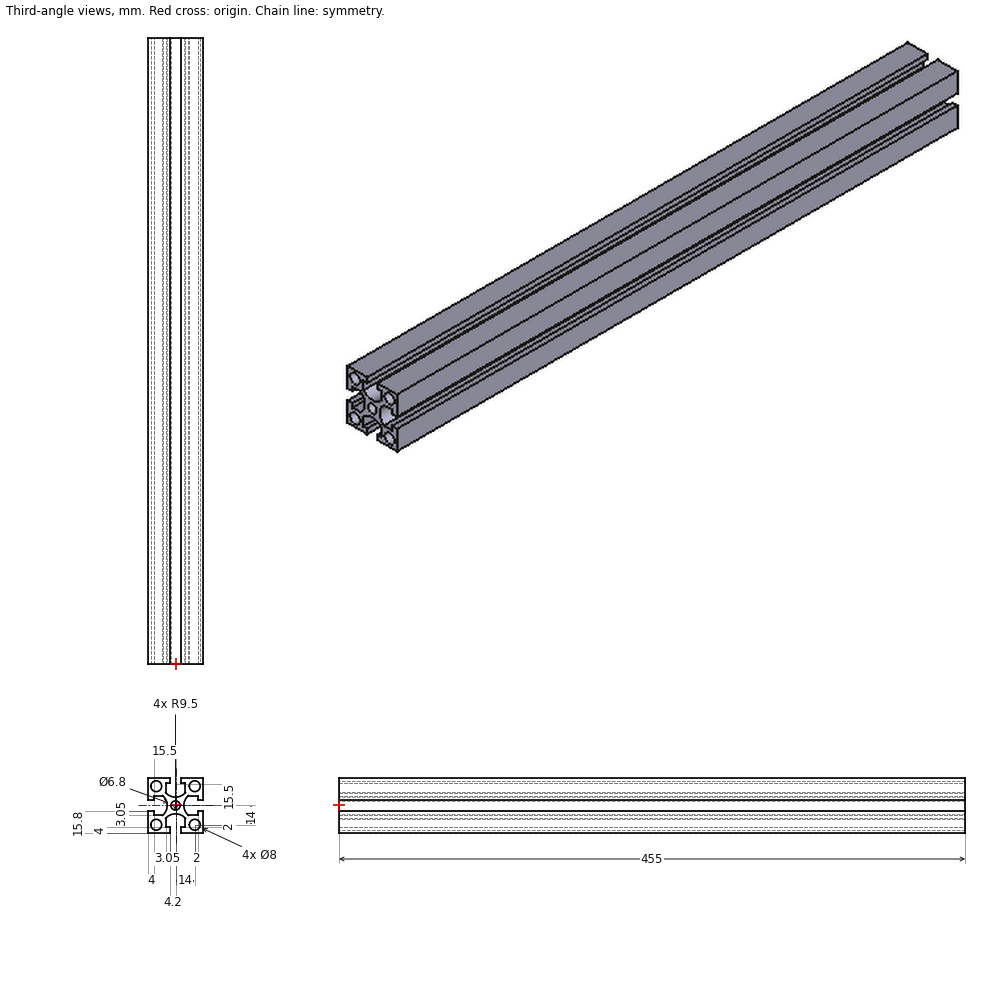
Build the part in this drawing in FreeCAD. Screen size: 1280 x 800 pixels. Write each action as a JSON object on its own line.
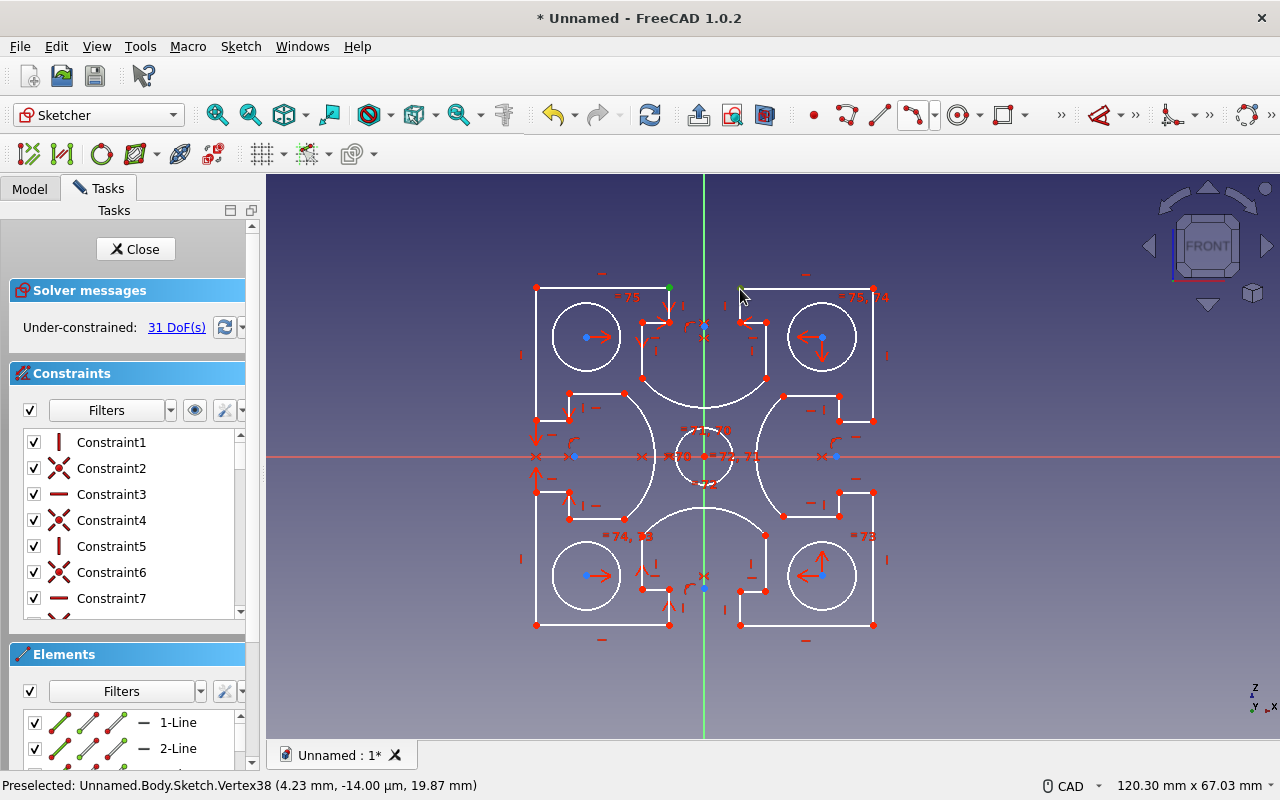
{"action": "left_click", "coordinate": [704, 675]}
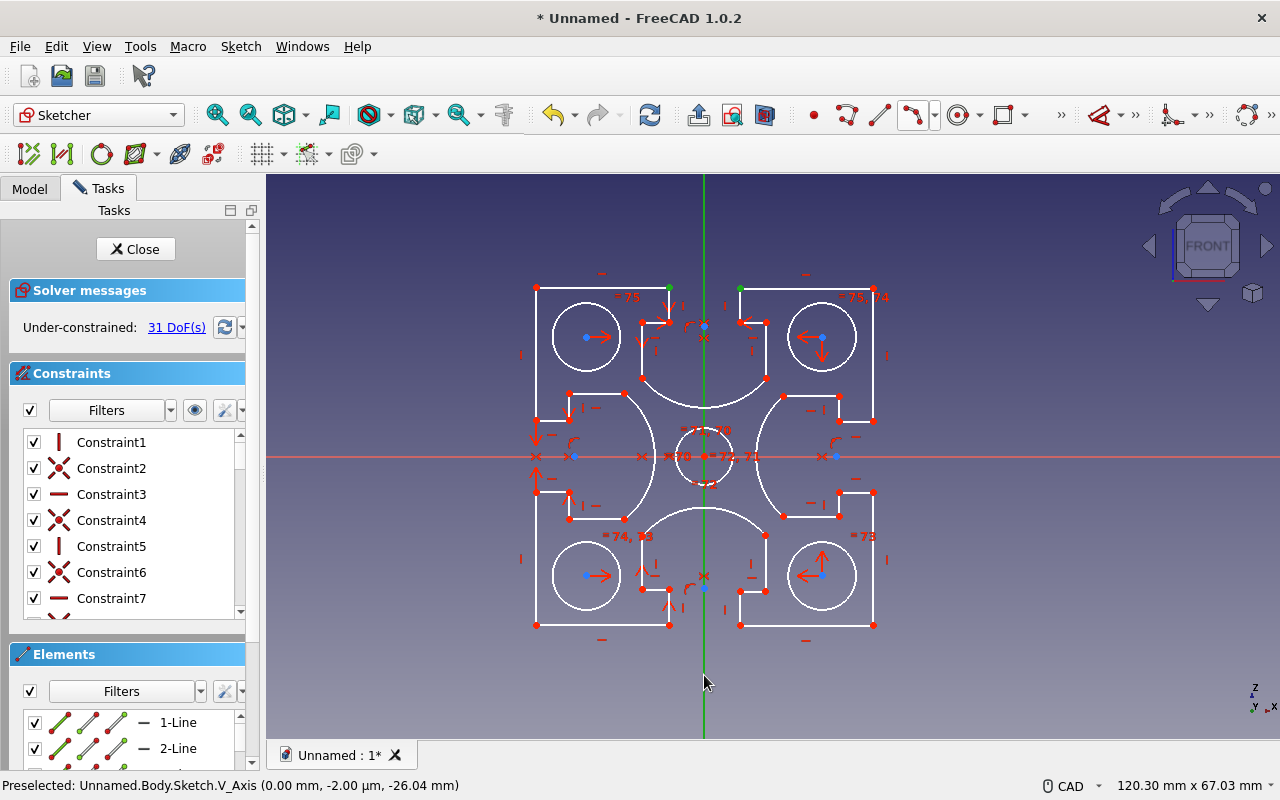
{"action": "key", "text": "s"}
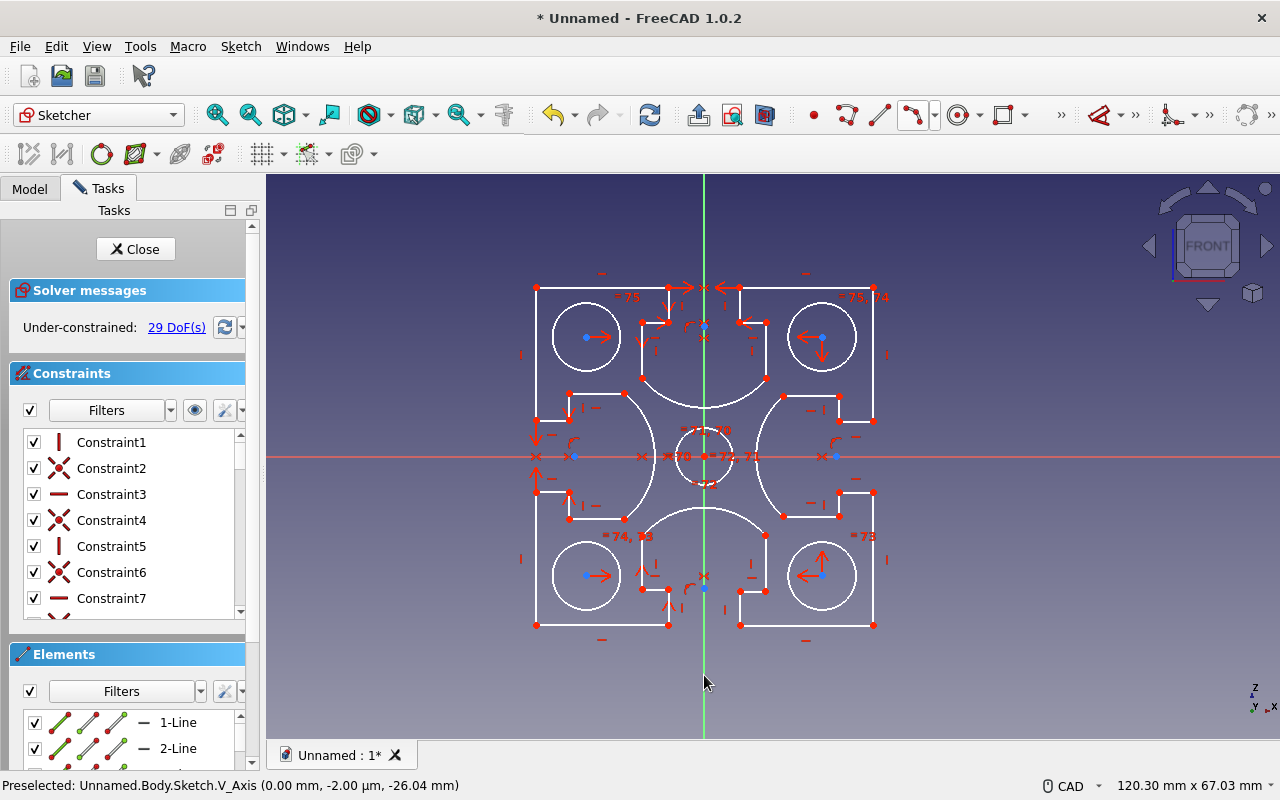
{"action": "left_click", "coordinate": [536, 421]}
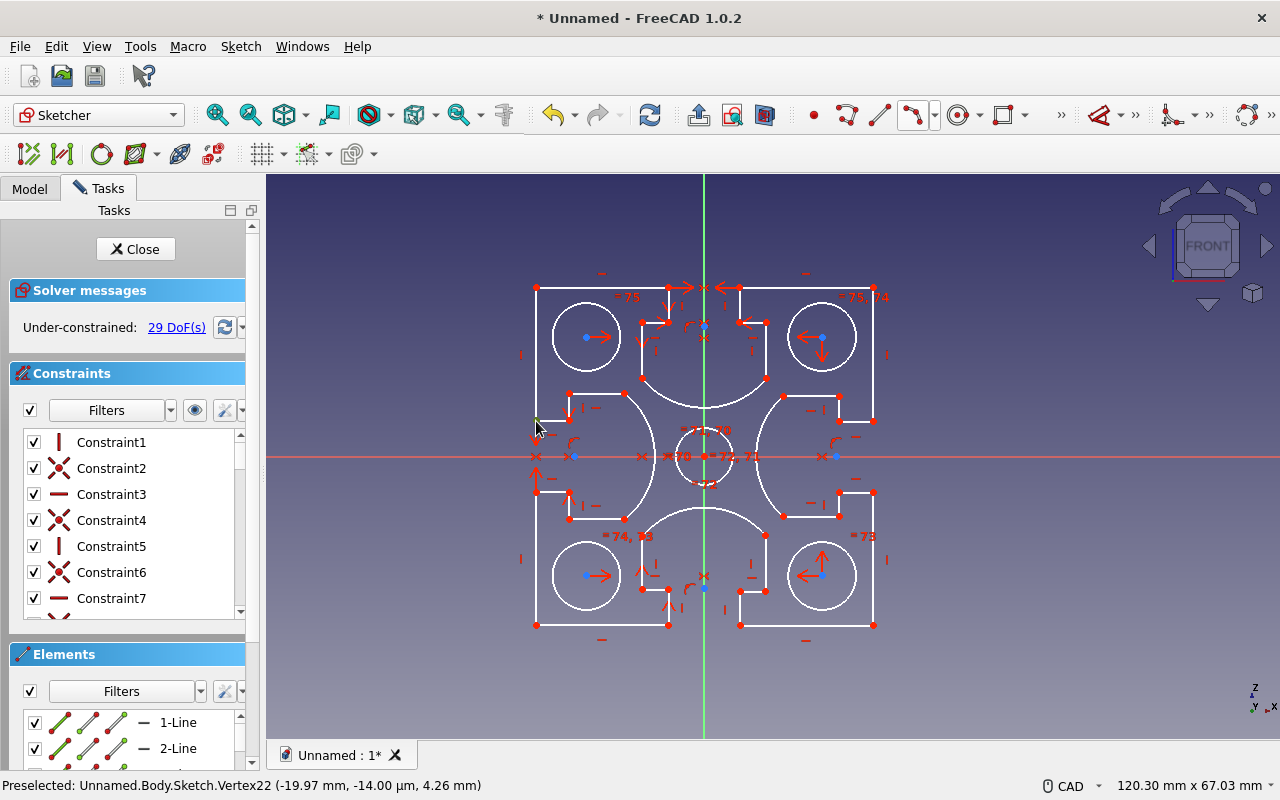
{"action": "left_click", "coordinate": [873, 422]}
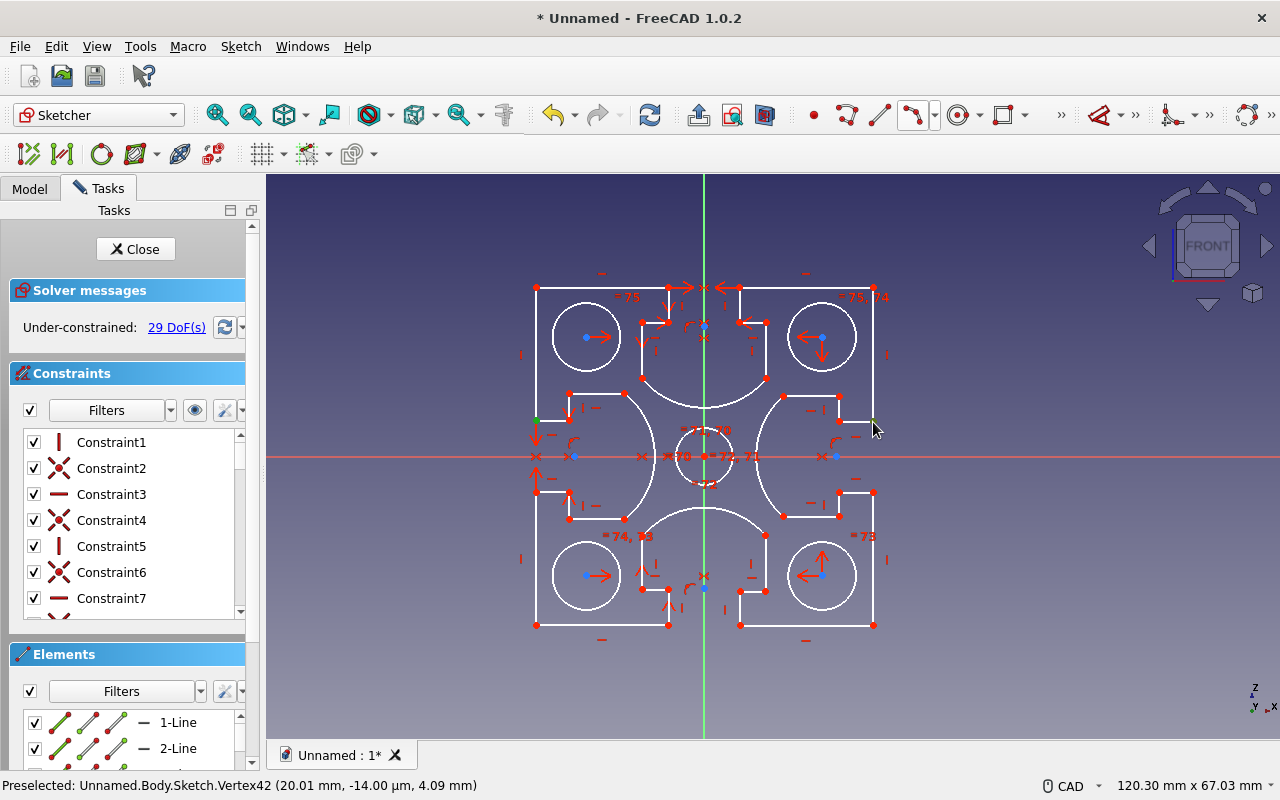
{"action": "left_click", "coordinate": [704, 675]}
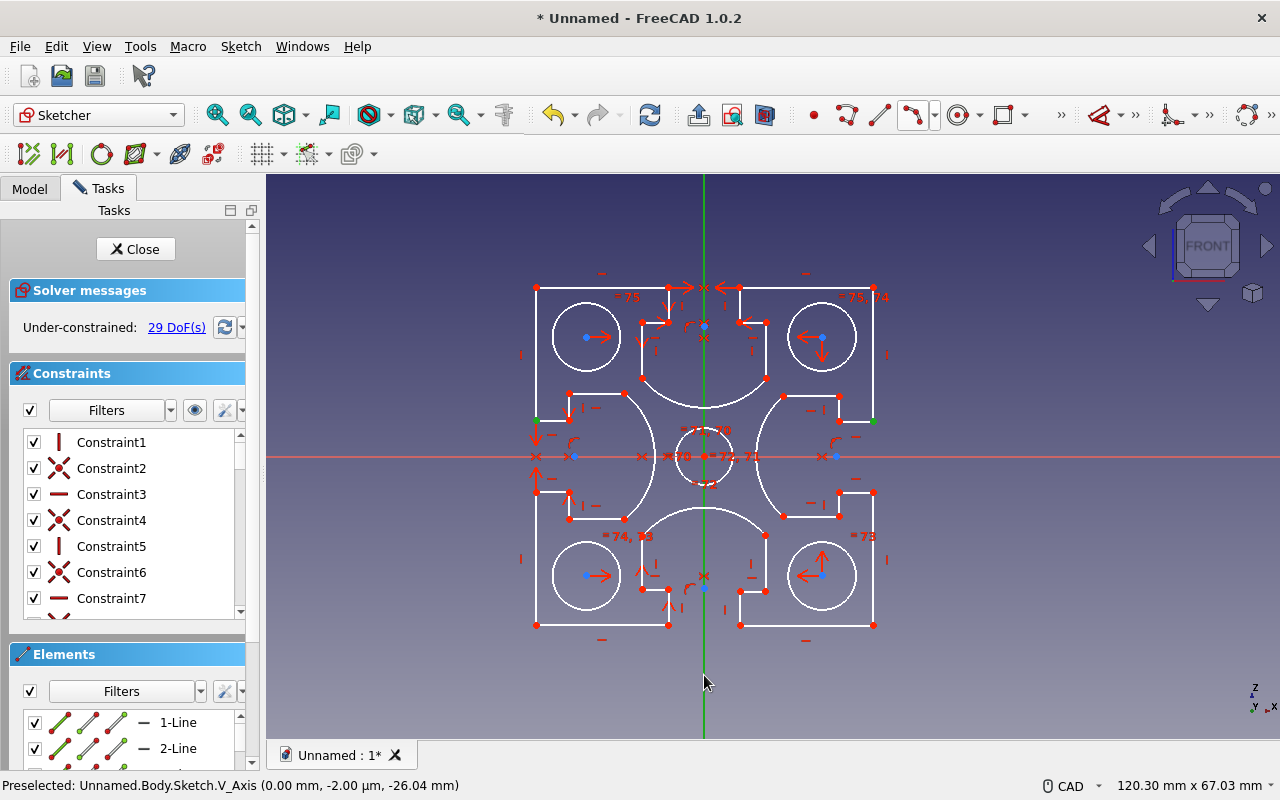
{"action": "key", "text": "s"}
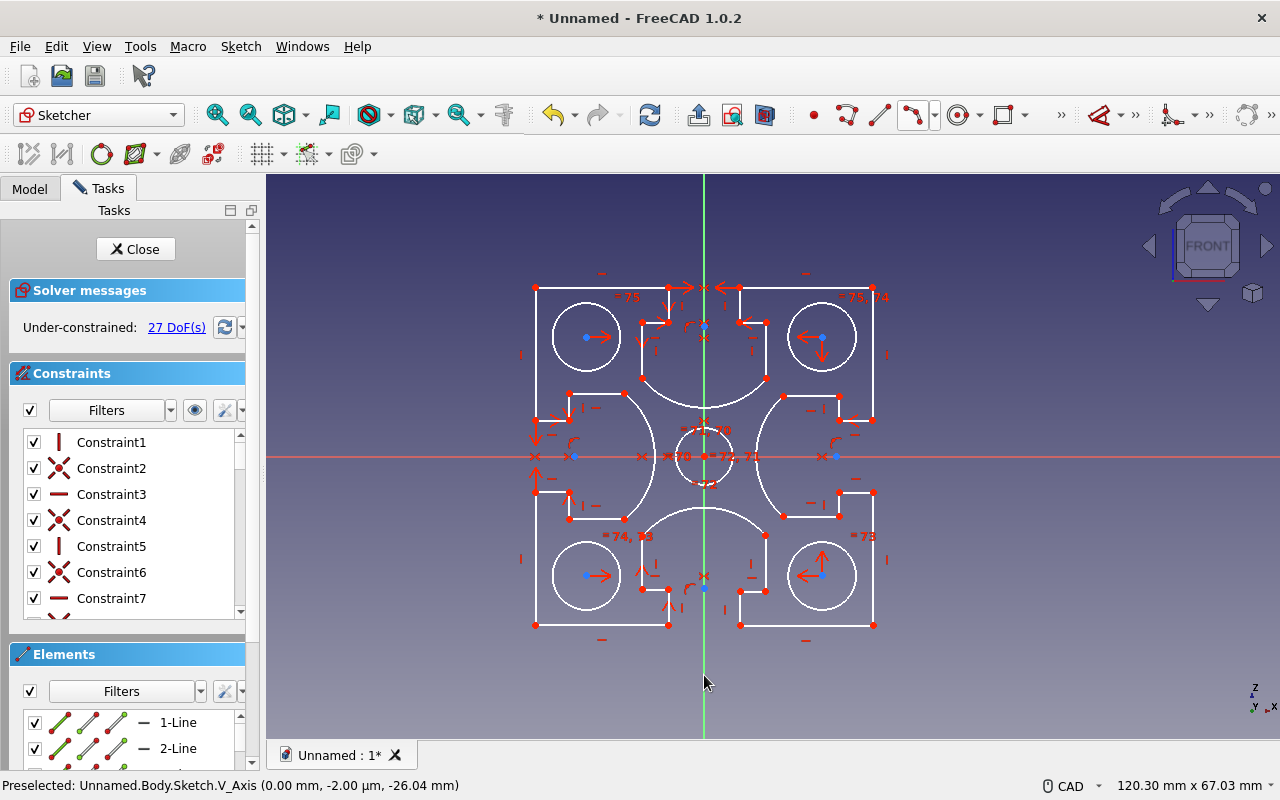
{"action": "left_click", "coordinate": [569, 394]}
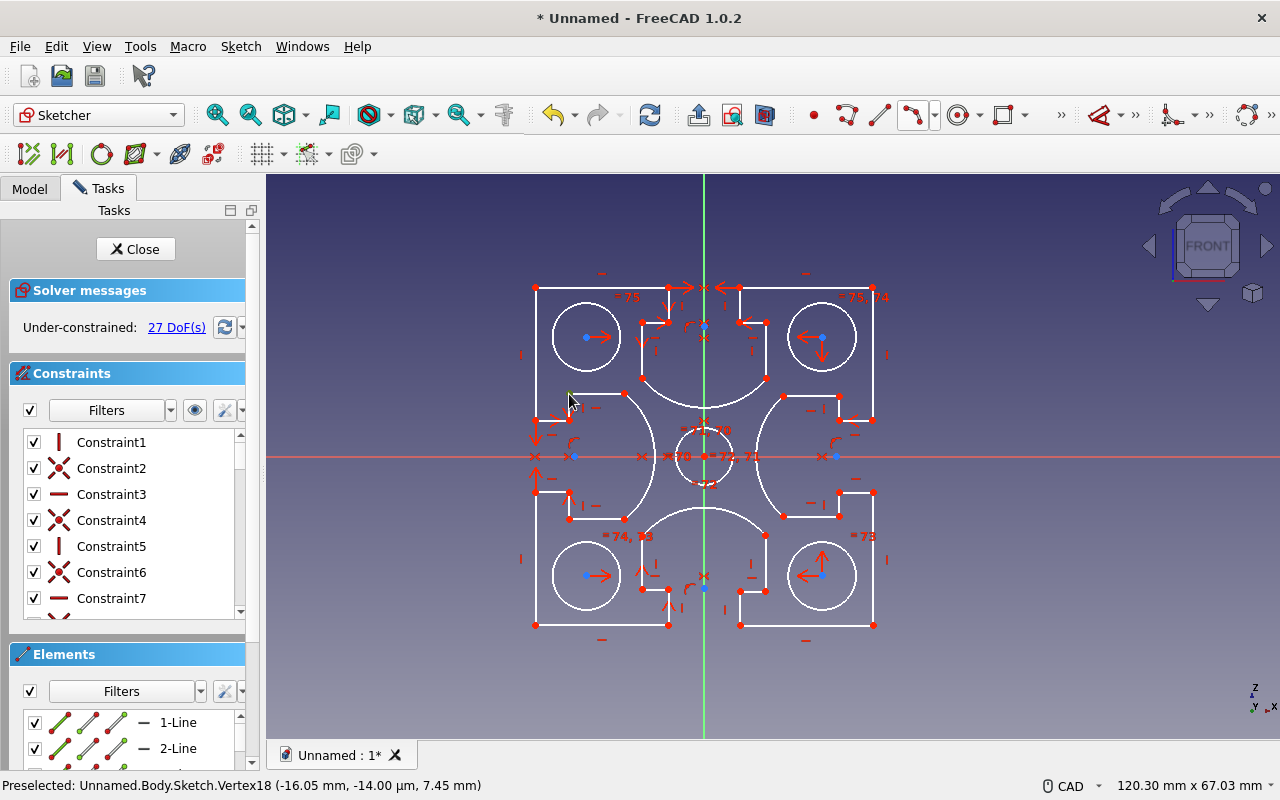
{"action": "left_click", "coordinate": [839, 396]}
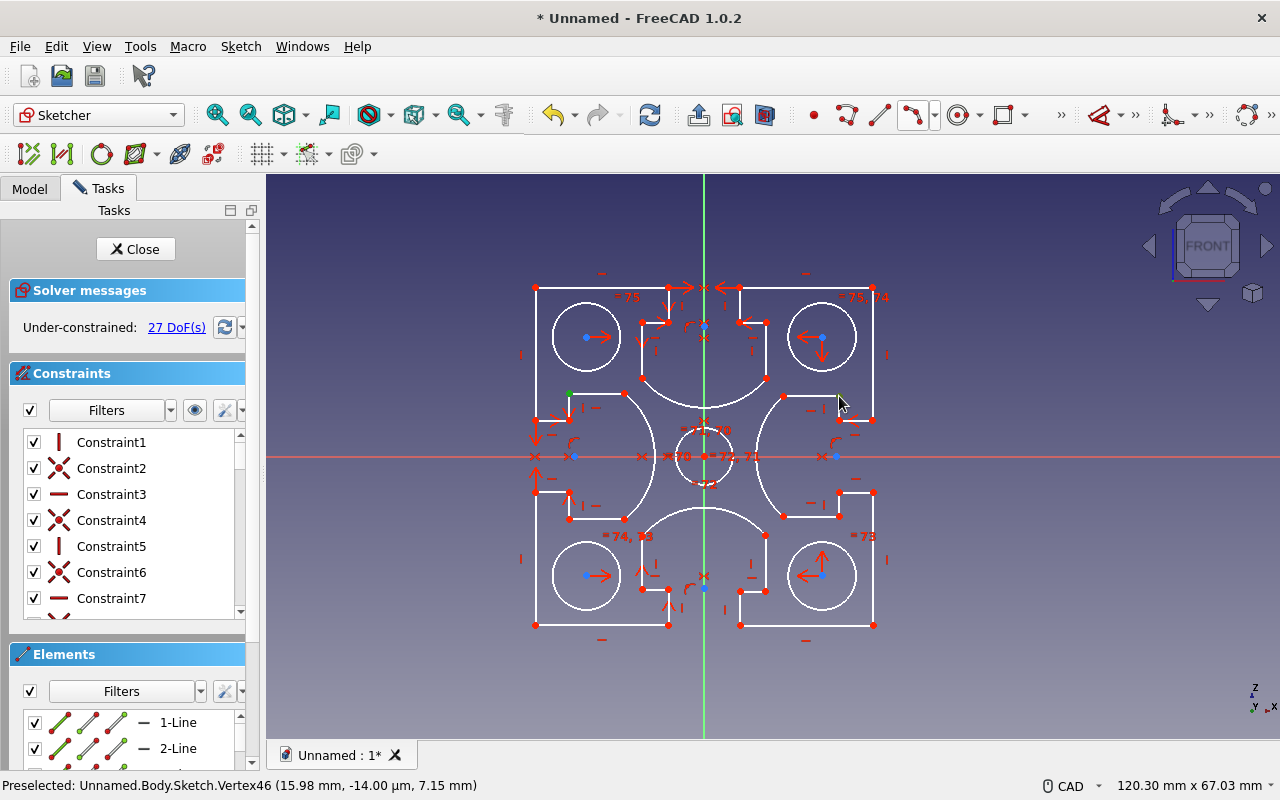
{"action": "left_click", "coordinate": [704, 675]}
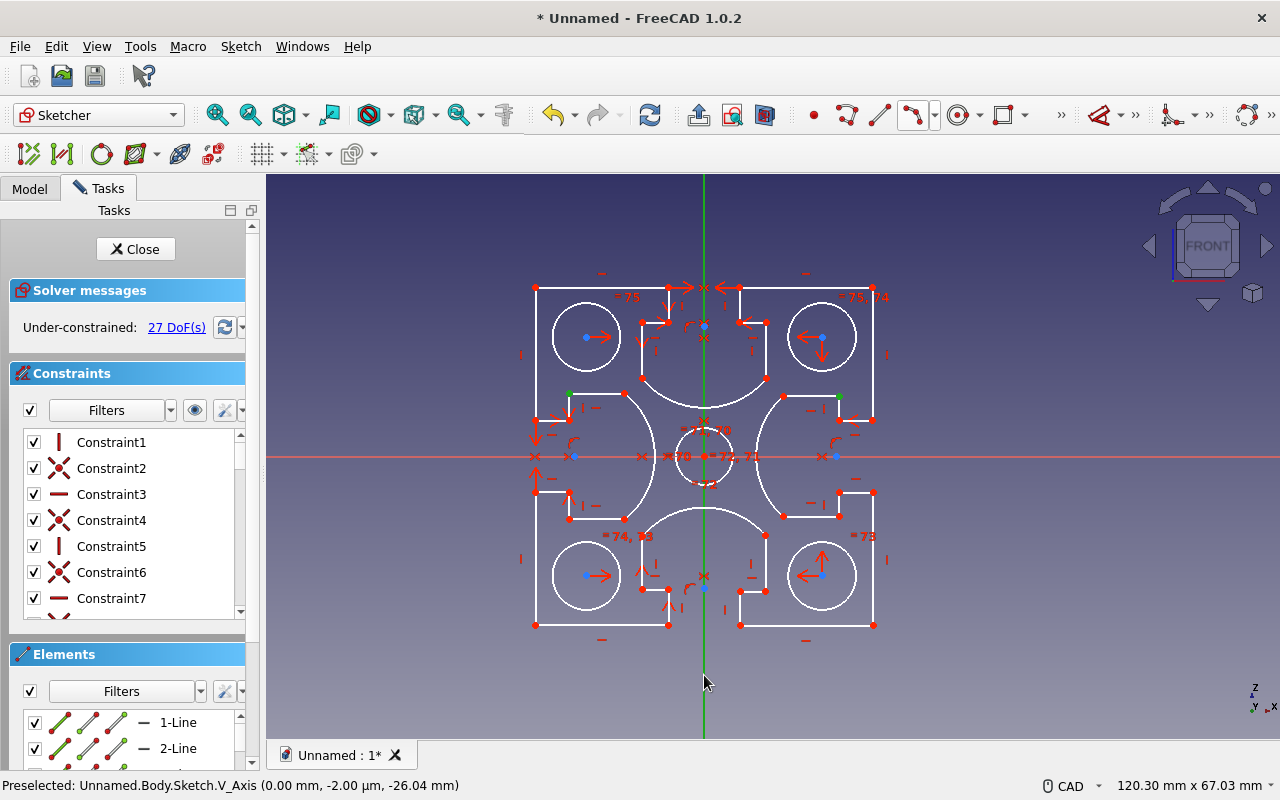
{"action": "key", "text": "s"}